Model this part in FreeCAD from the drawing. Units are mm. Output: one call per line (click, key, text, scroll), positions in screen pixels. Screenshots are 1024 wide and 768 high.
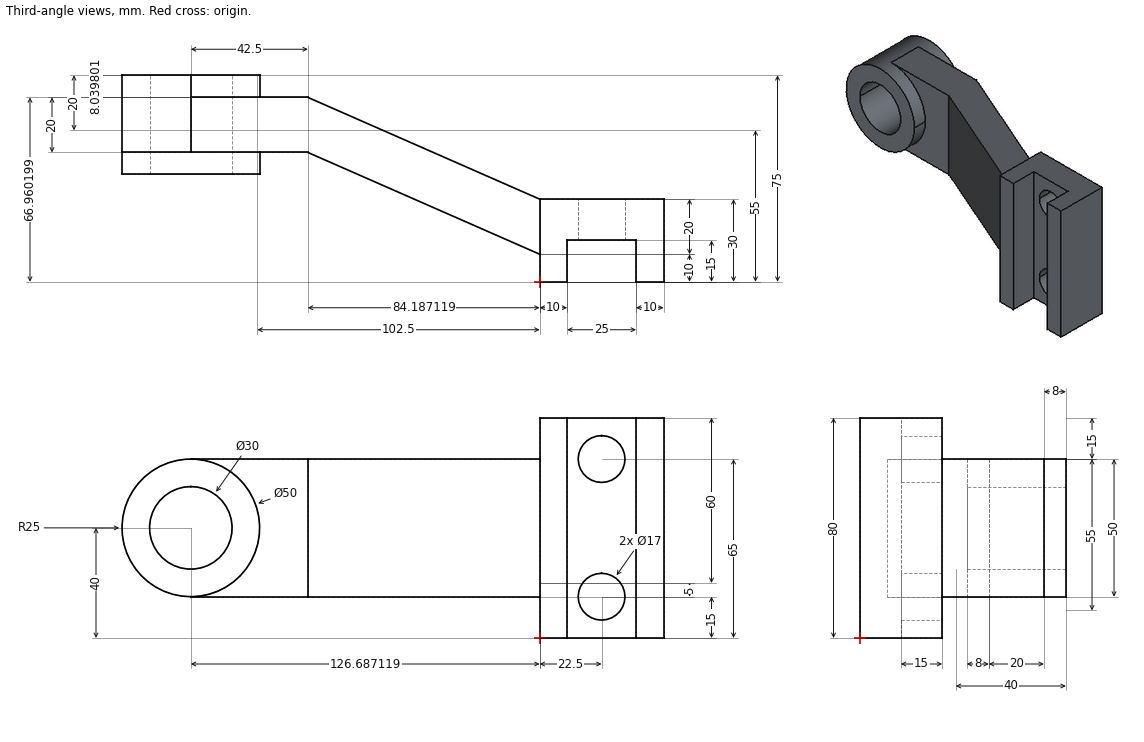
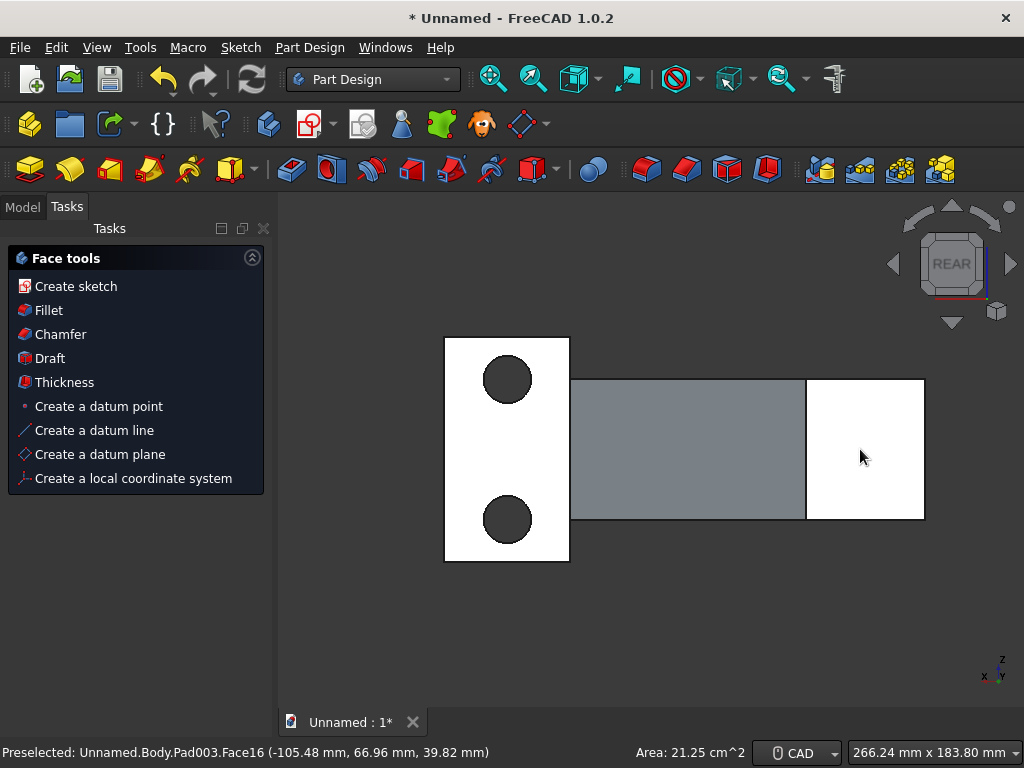
click(310, 124)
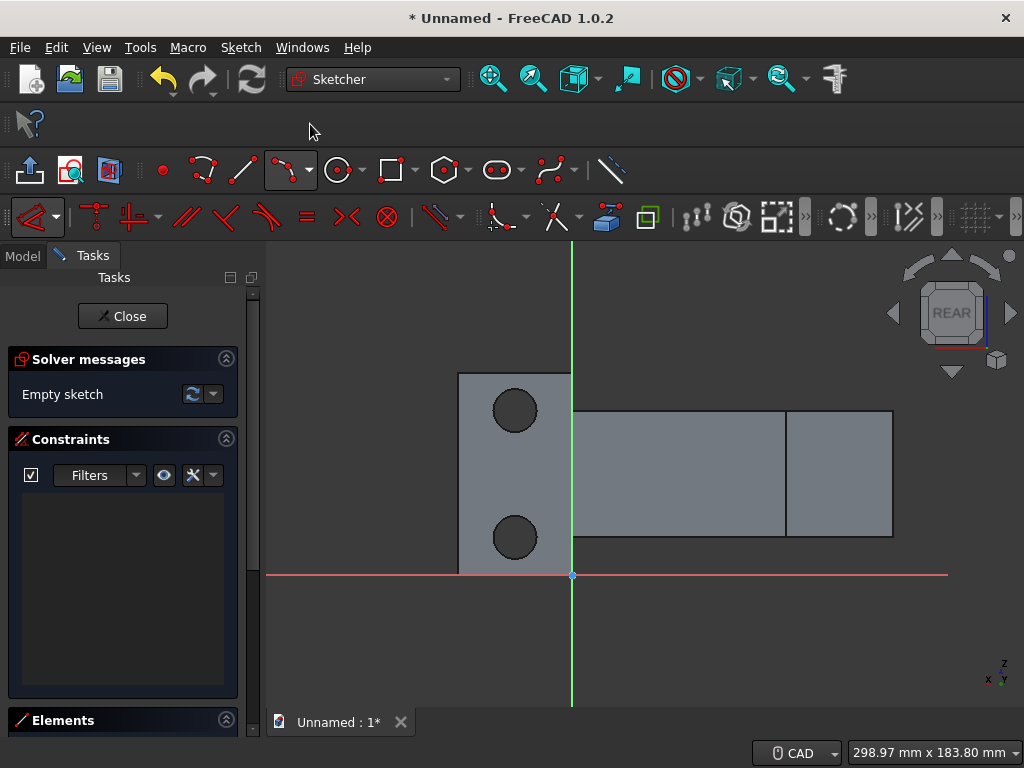
scroll(576, 474, down, 5)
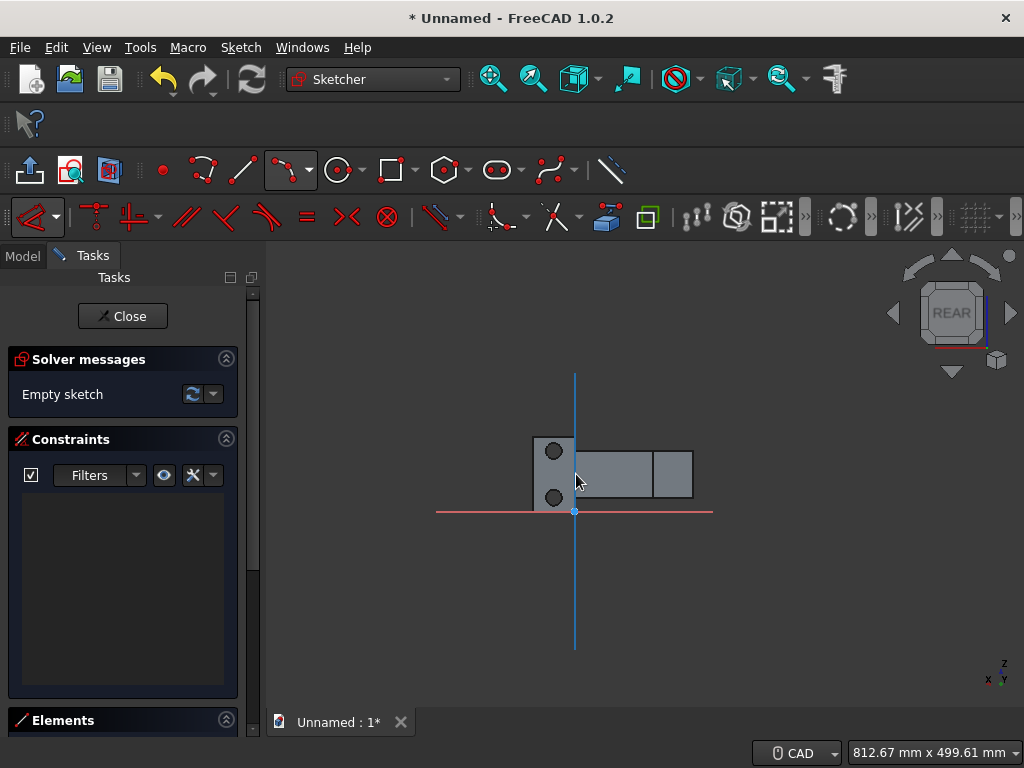
scroll(716, 474, up, 9)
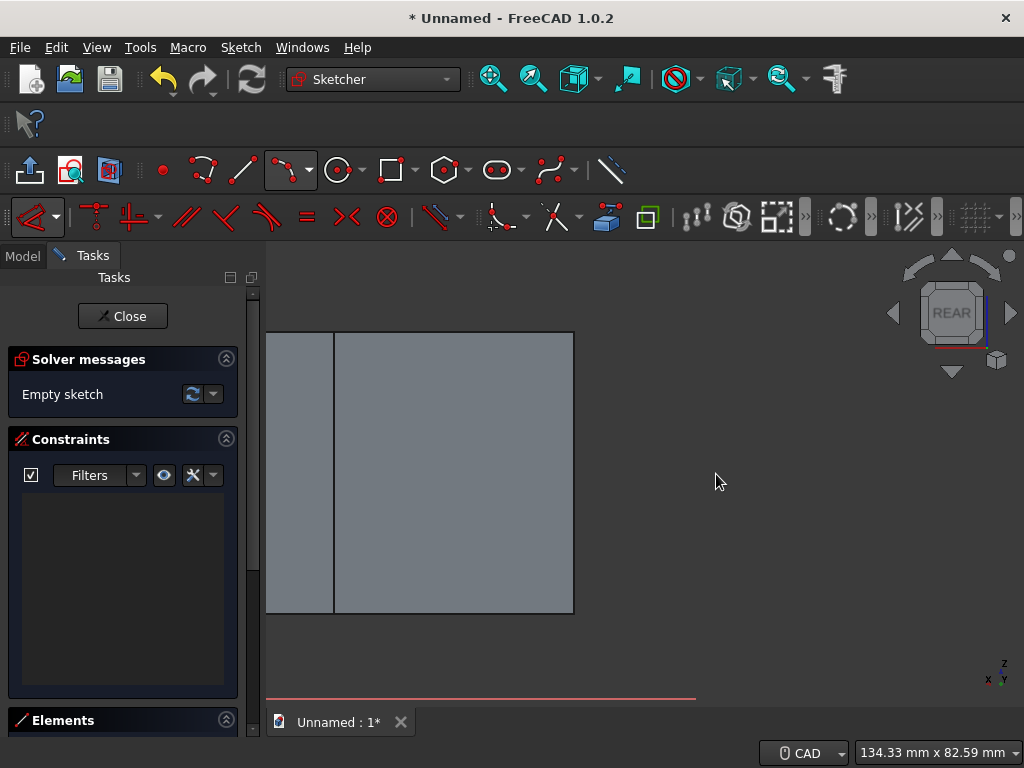
click(338, 170)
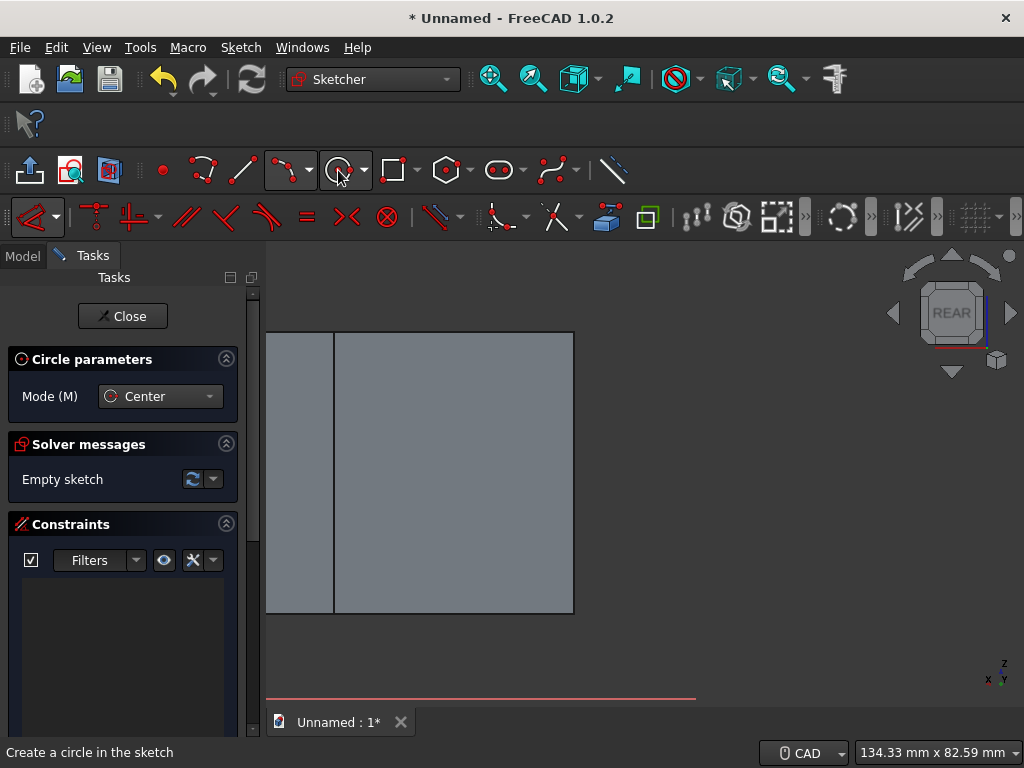
click(574, 473)
move(674, 374)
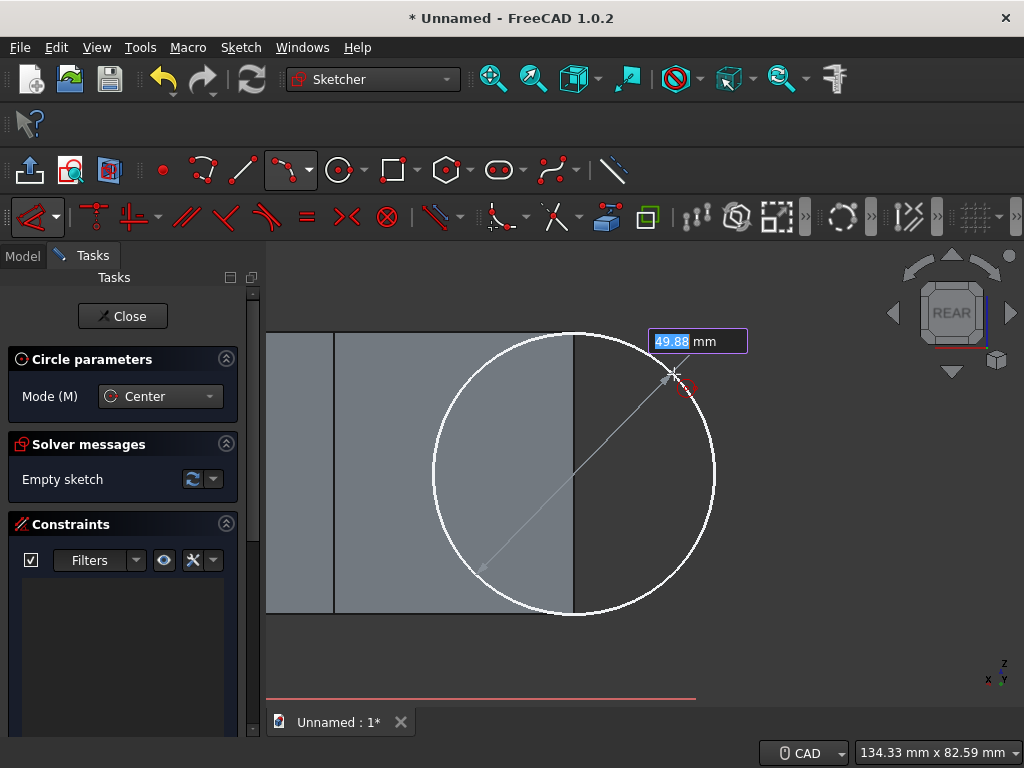
text(50)
key(Return)
key(Escape)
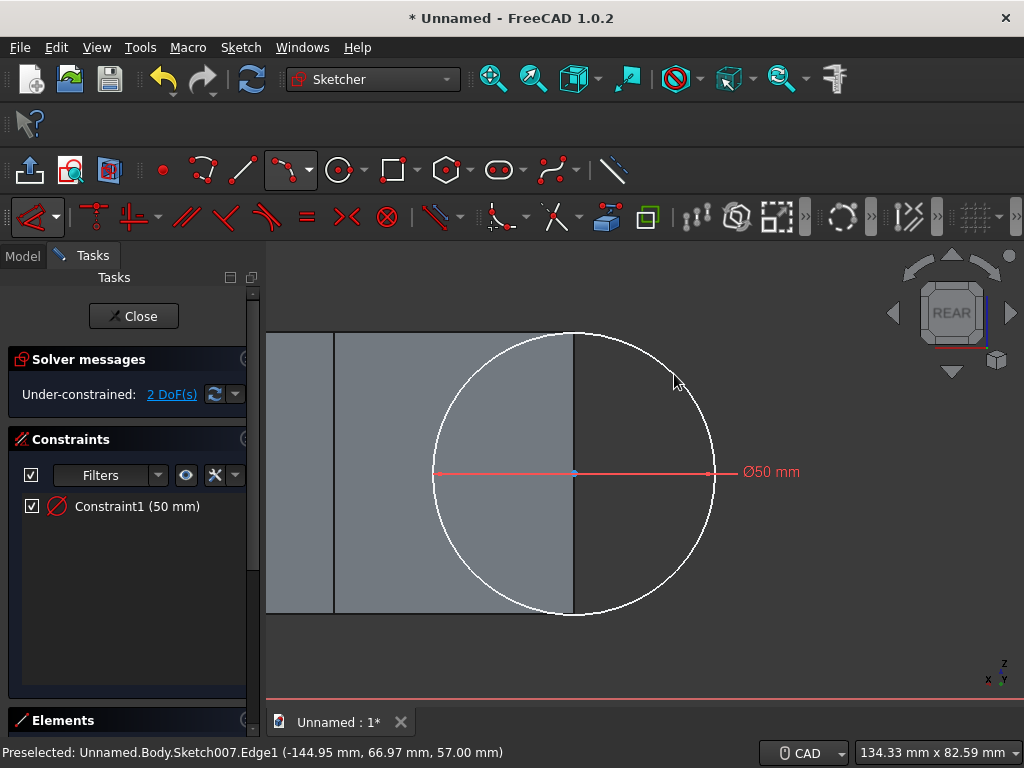
click(574, 474)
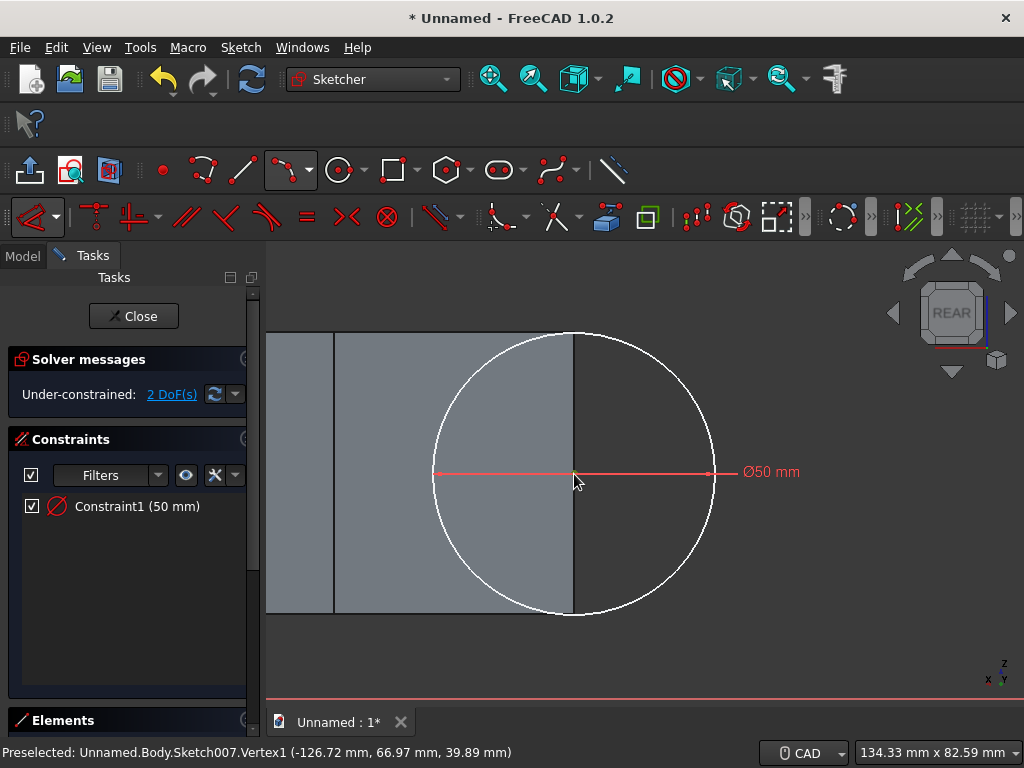
key(i)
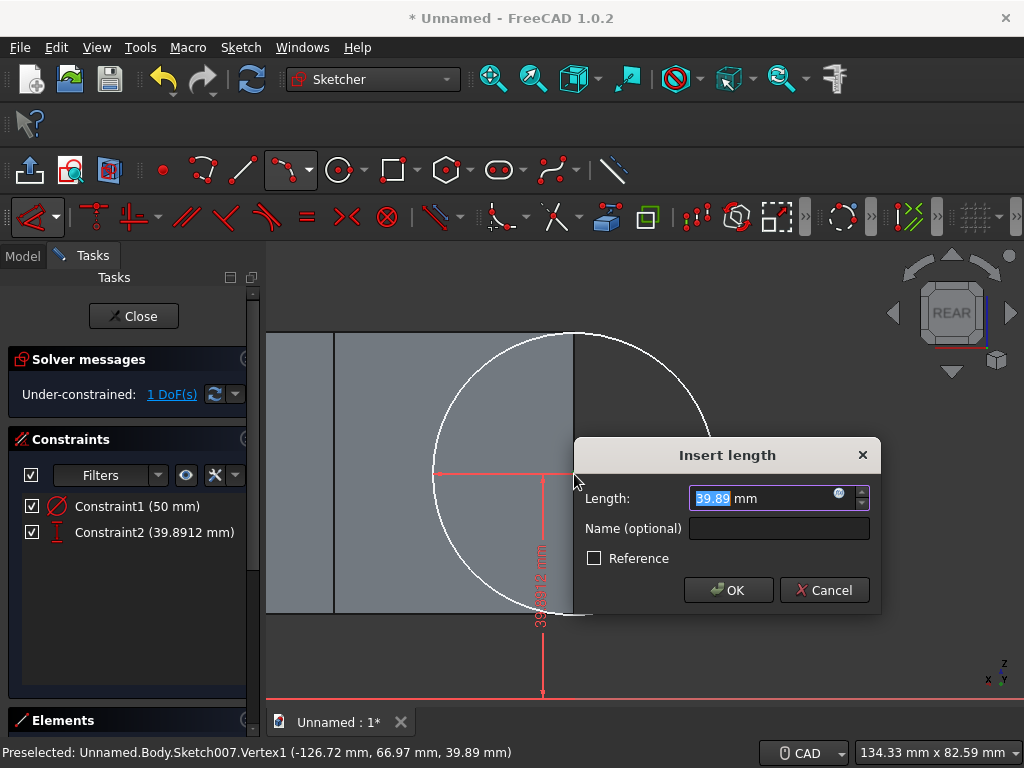
text(40)
key(Return)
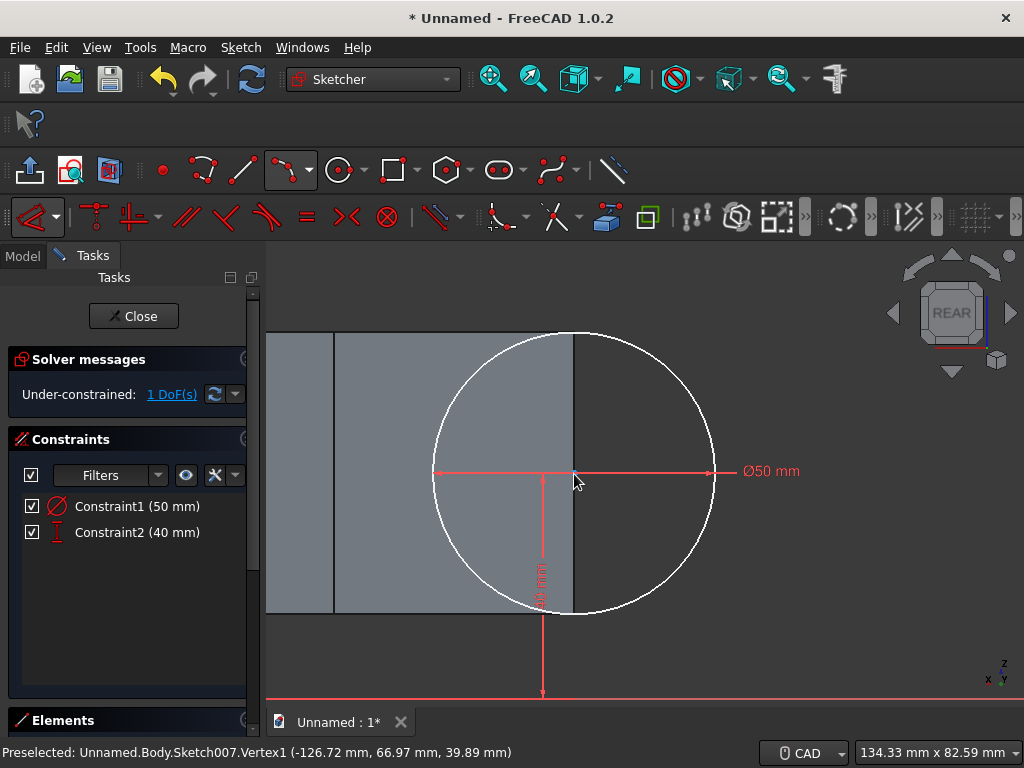
click(574, 473)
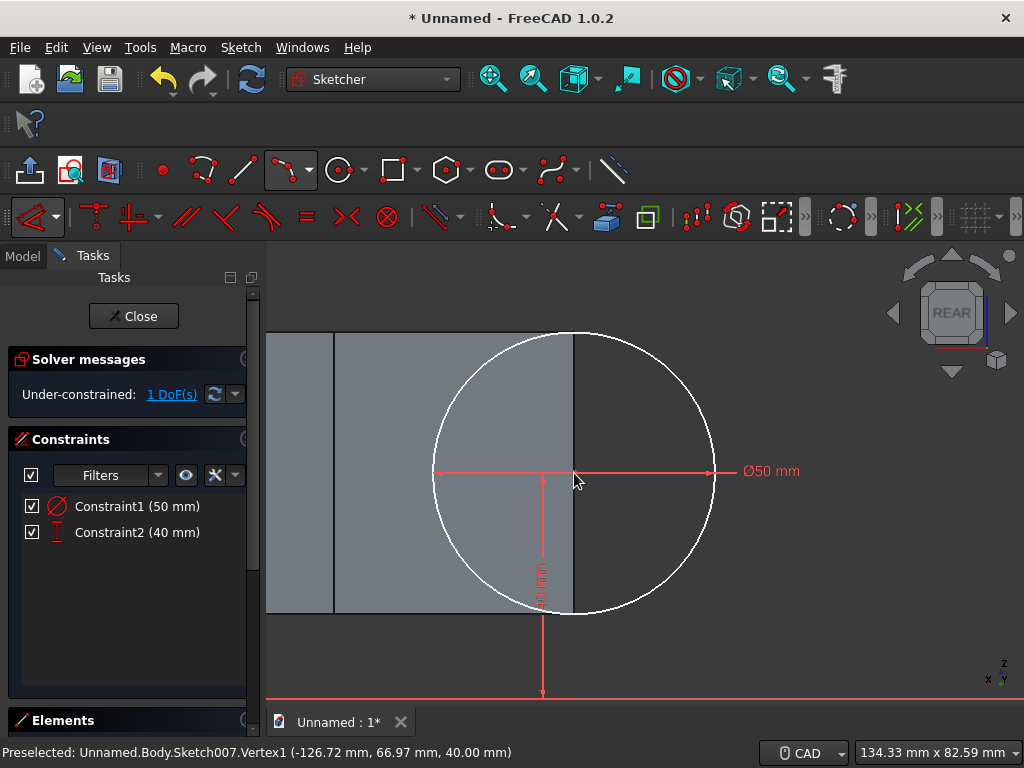
click(58, 218)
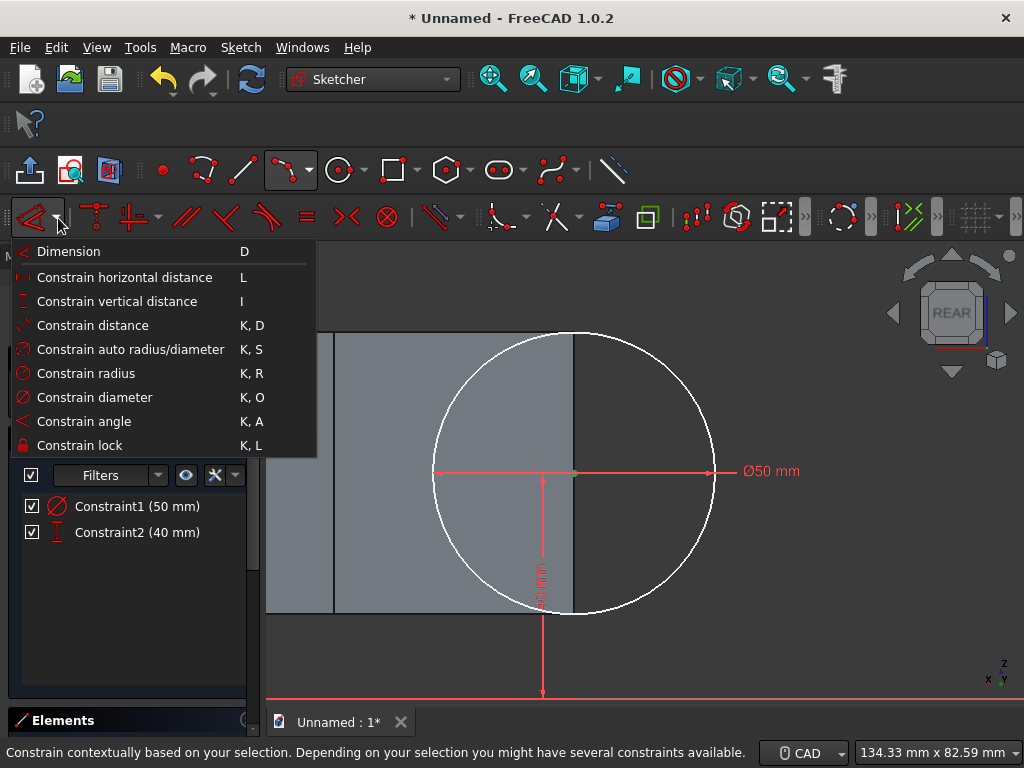
click(164, 277)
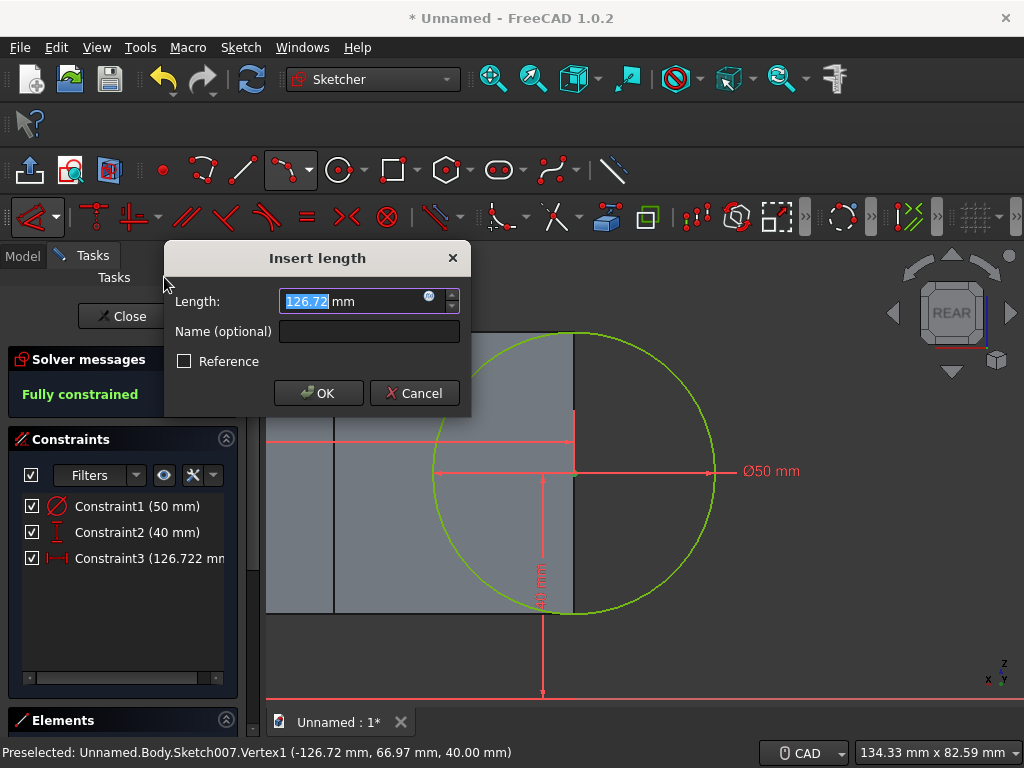
text(126.687119)
key(Return)